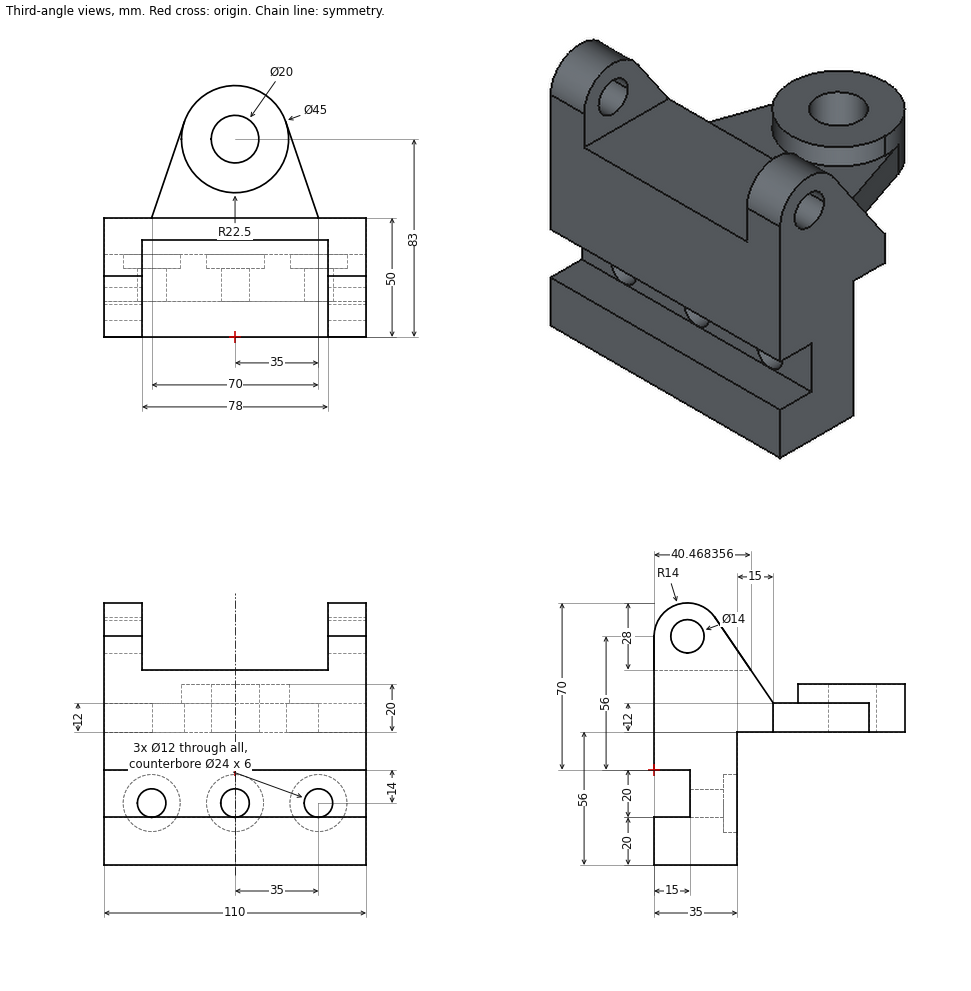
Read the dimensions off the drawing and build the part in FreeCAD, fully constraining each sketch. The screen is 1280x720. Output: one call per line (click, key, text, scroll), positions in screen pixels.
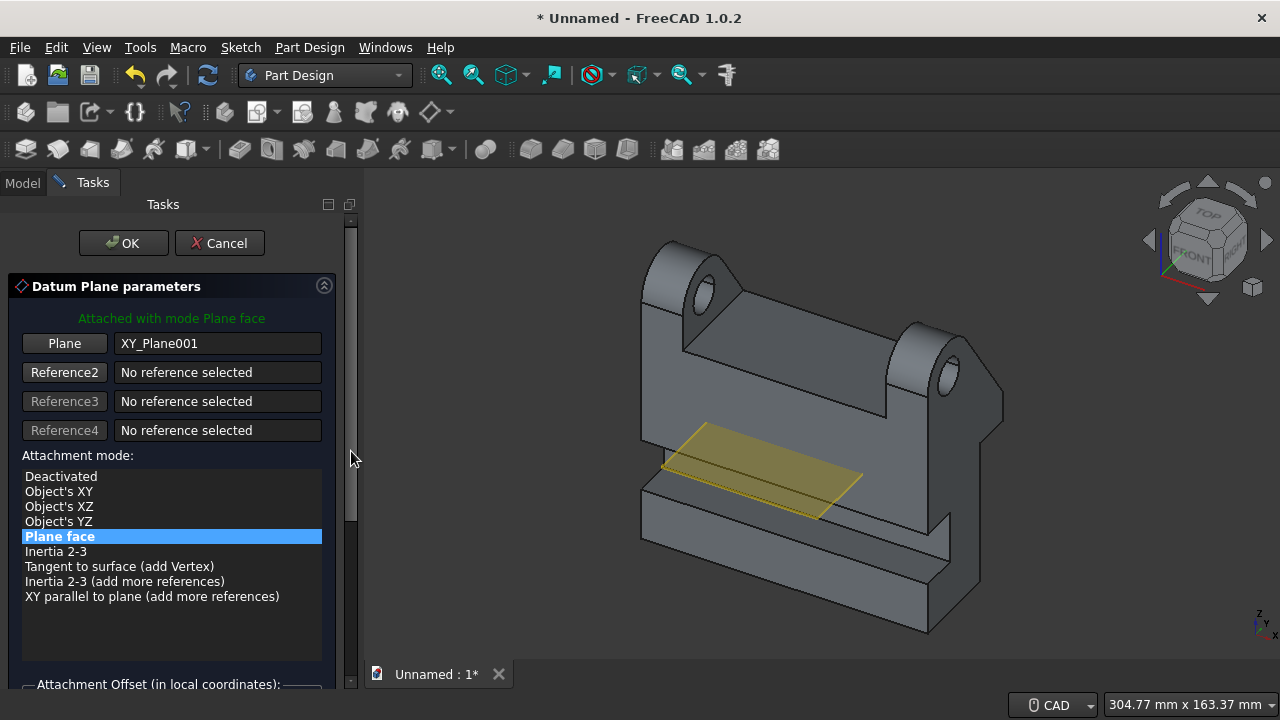
click(124, 243)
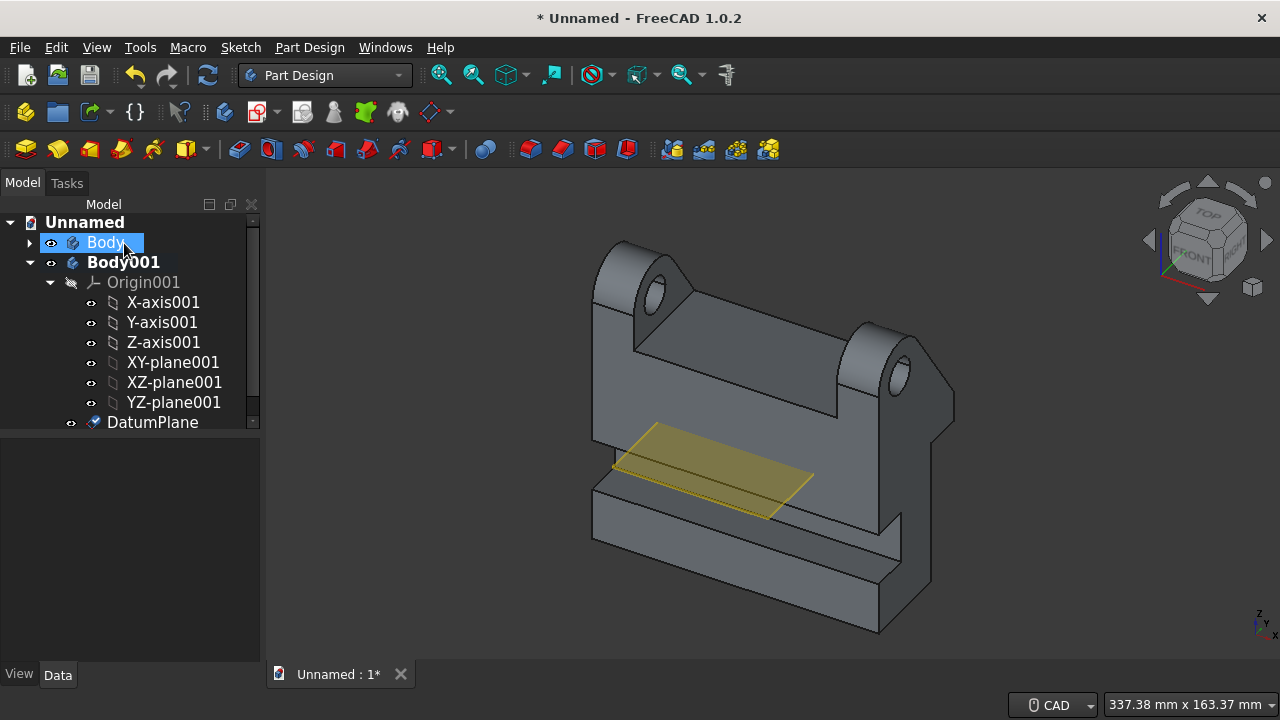
click(116, 423)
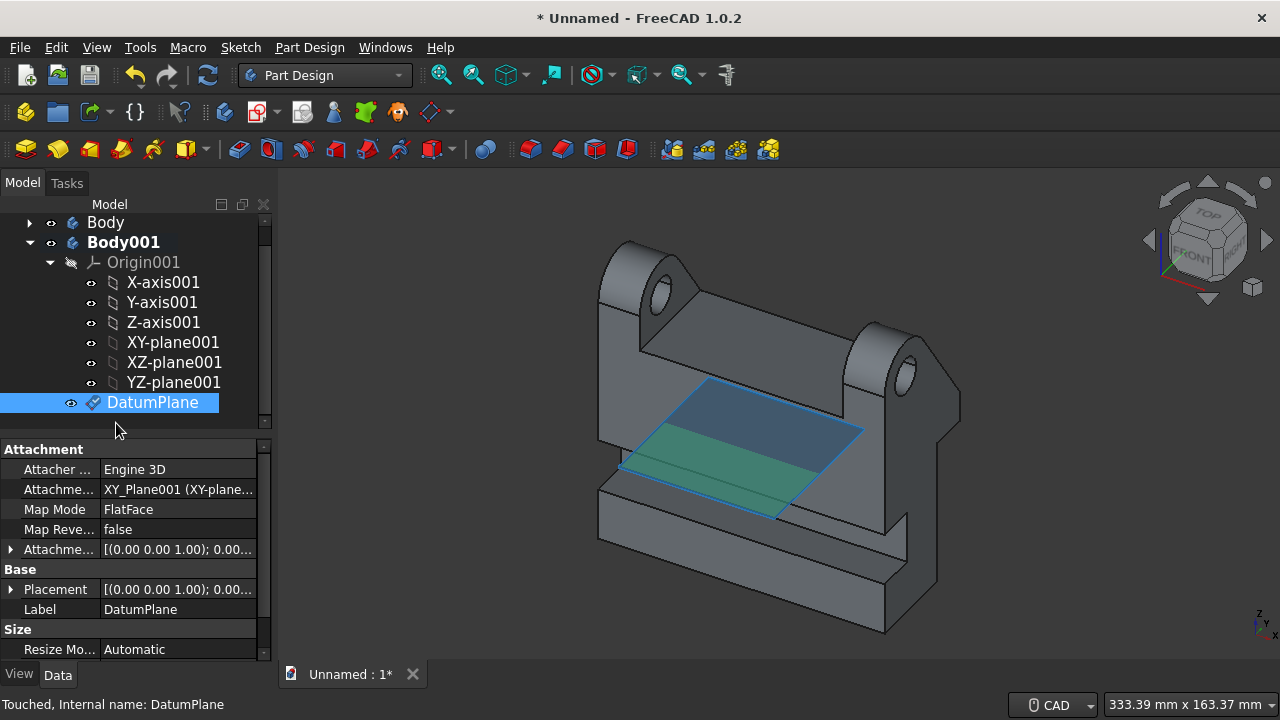
click(258, 112)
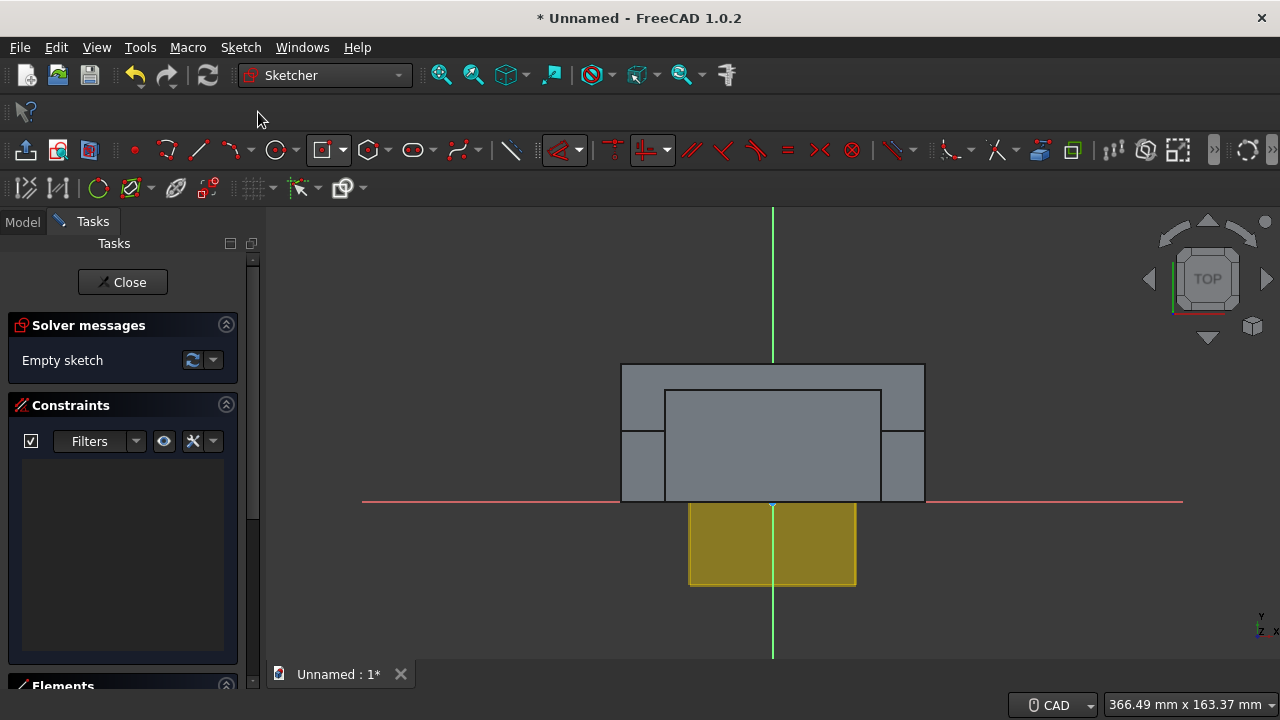
scroll(395, 631, down, 1)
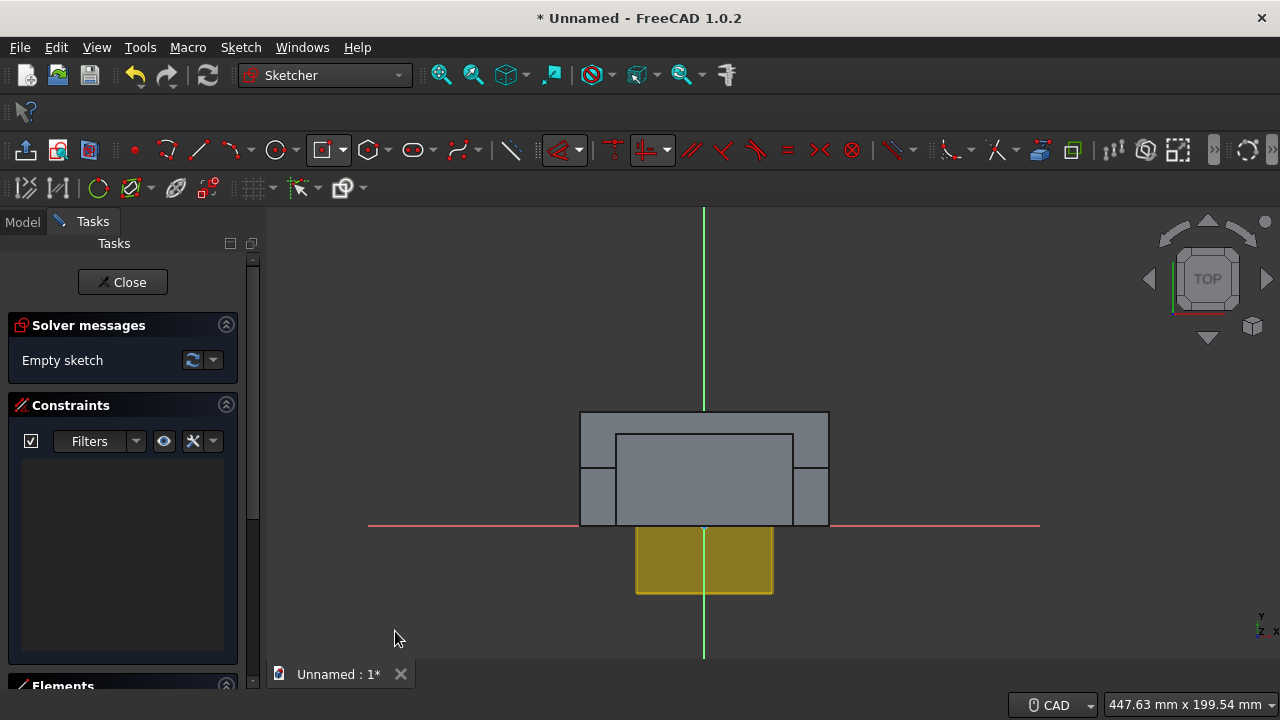
click(276, 150)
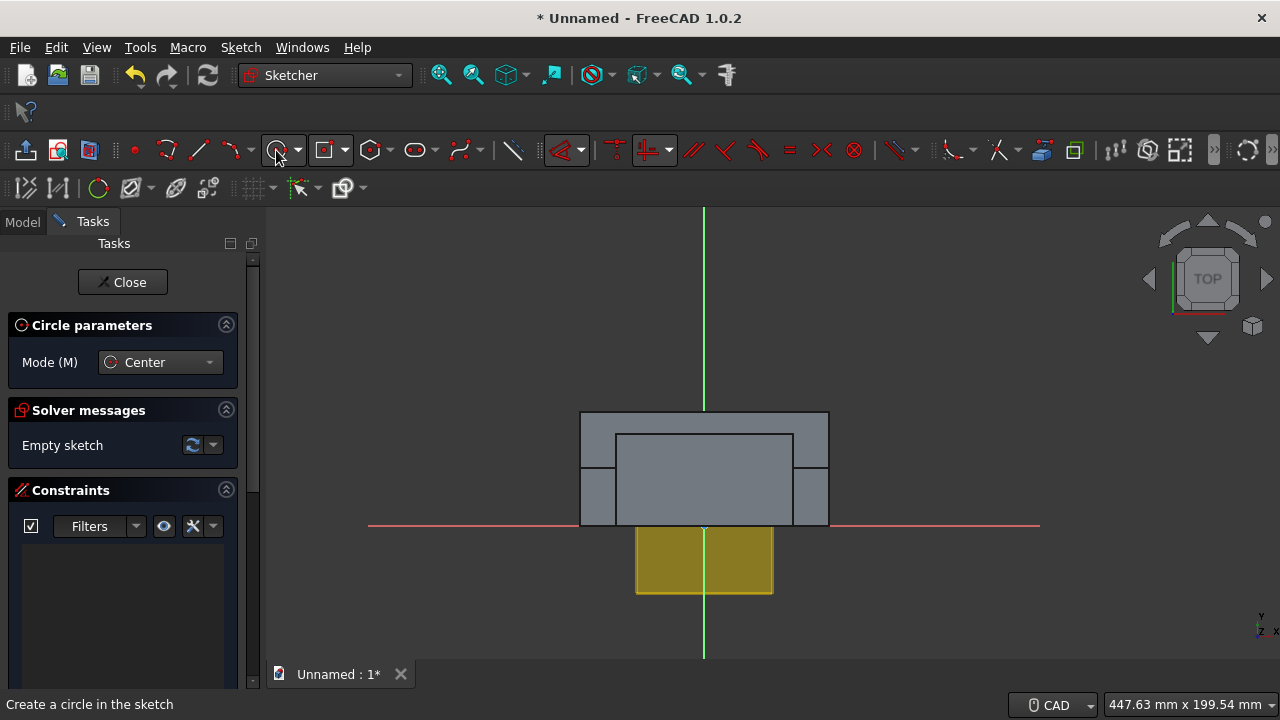
click(704, 338)
click(741, 302)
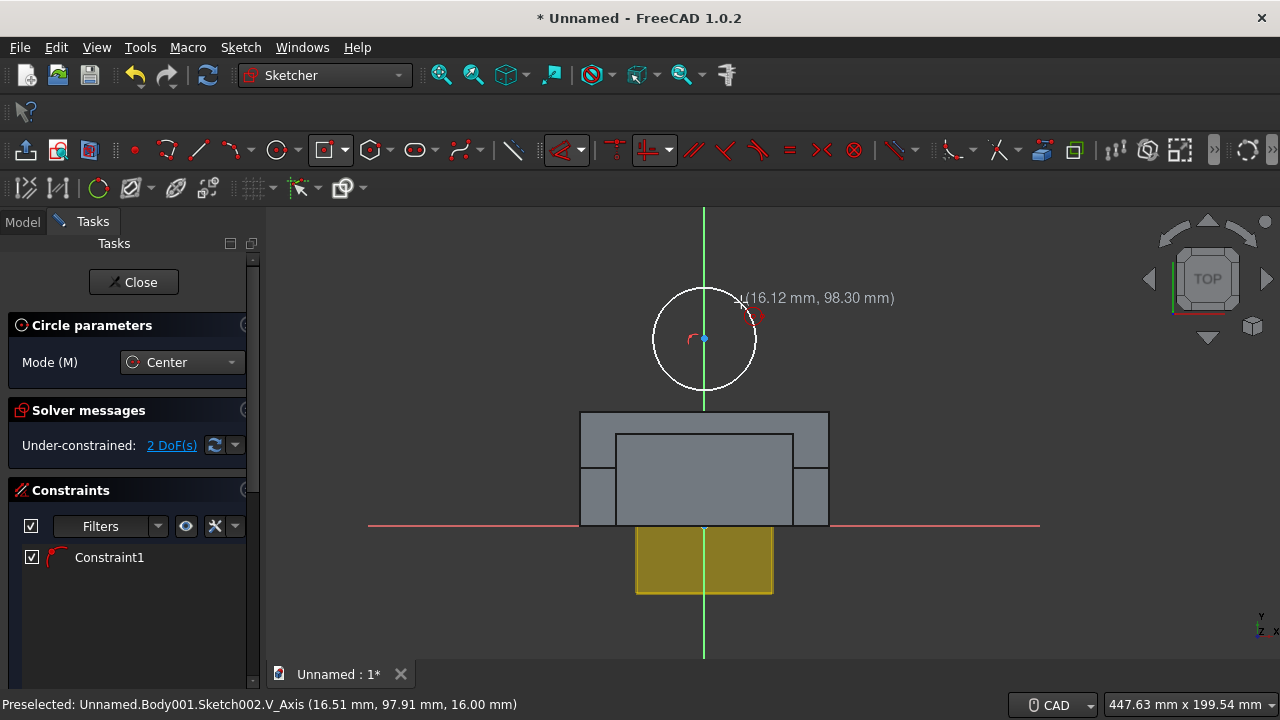
click(704, 339)
click(721, 322)
key(Escape)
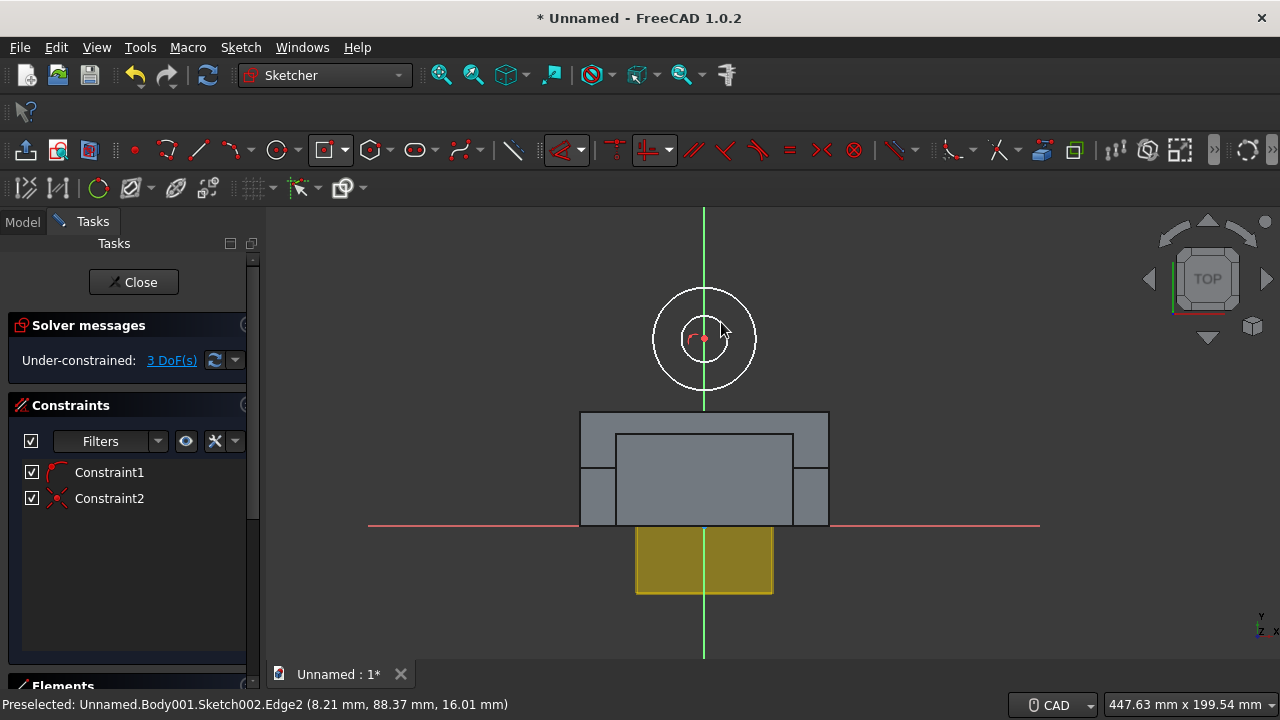
click(741, 303)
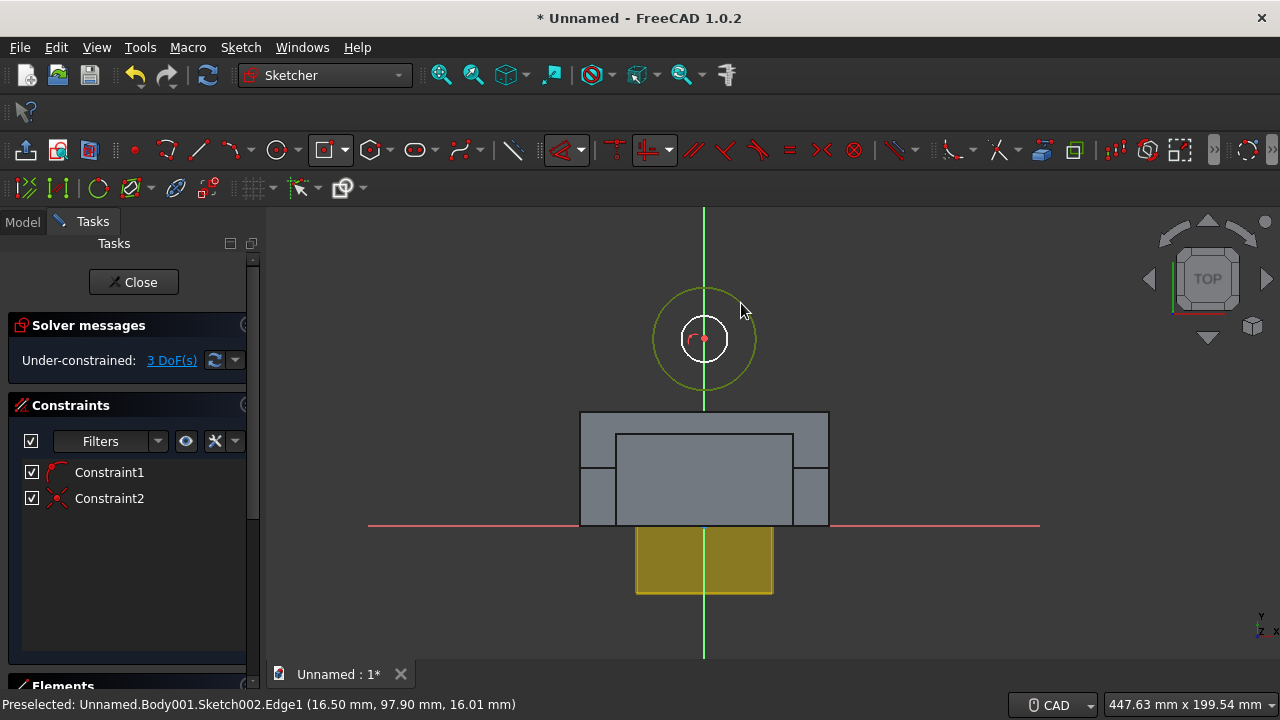
key(k)
key(o)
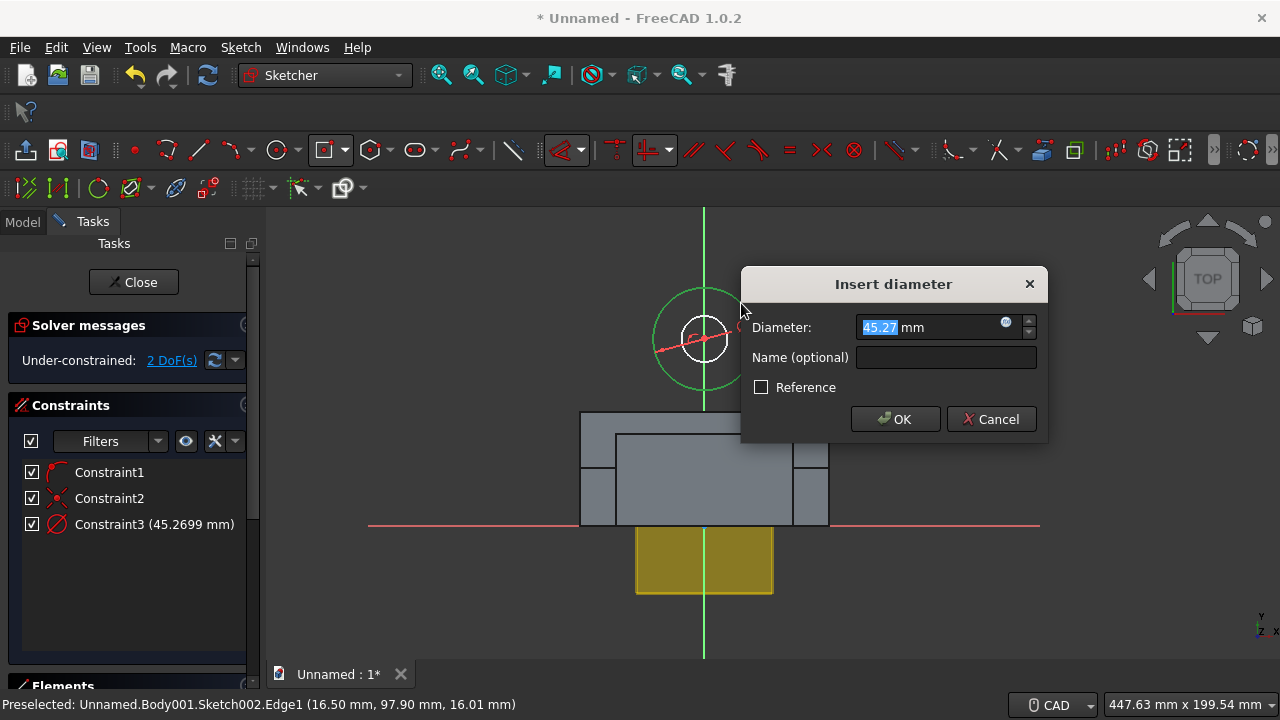
text(45)
key(Return)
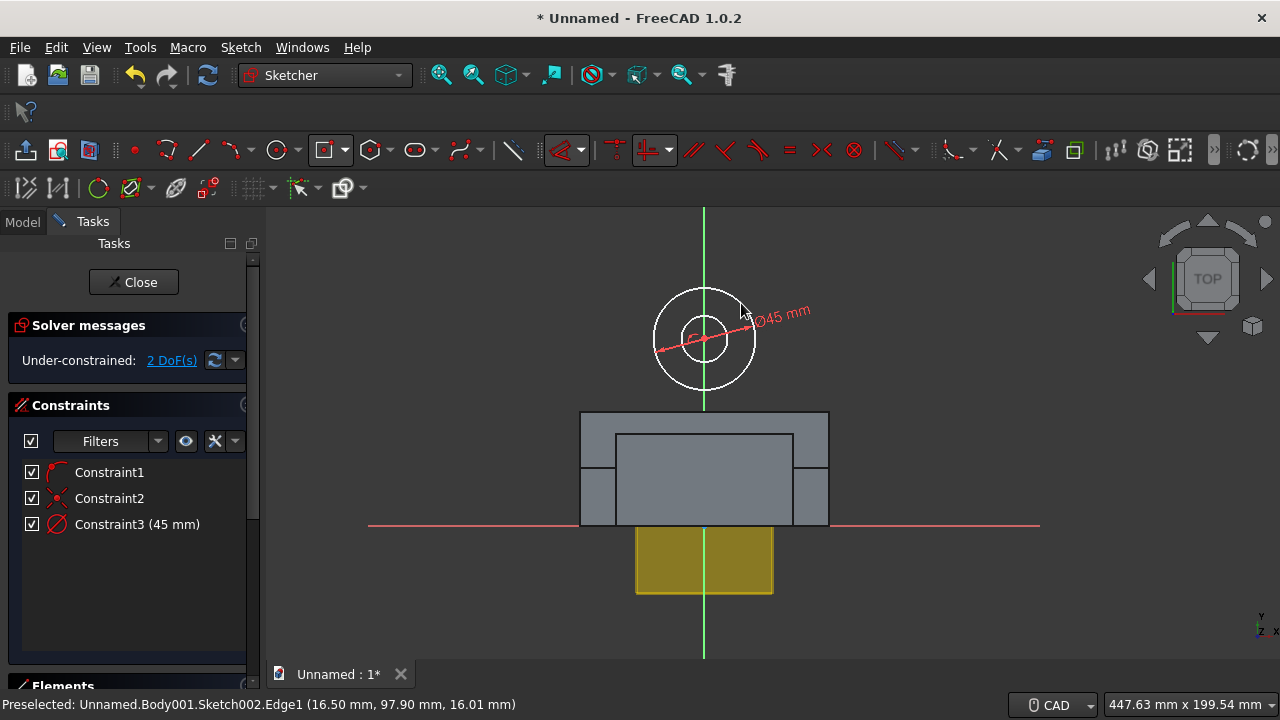
click(721, 323)